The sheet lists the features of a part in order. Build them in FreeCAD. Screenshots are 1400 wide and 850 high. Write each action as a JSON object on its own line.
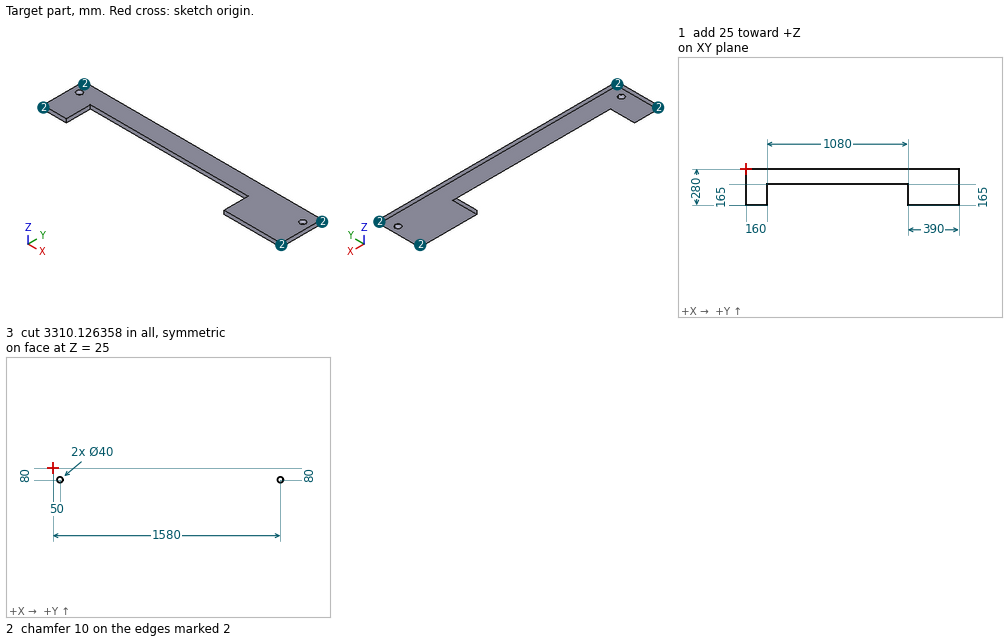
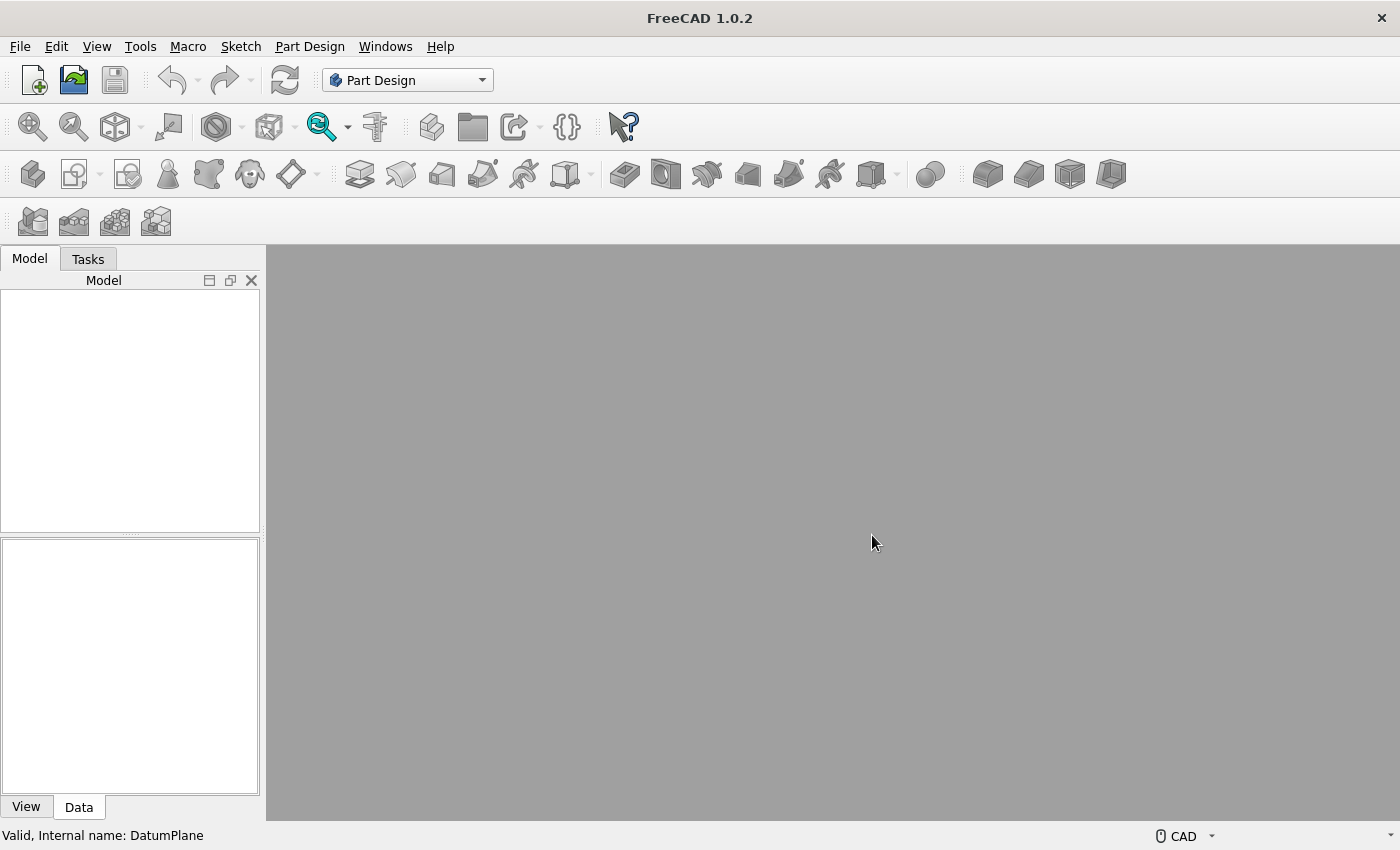
{"action": "key", "text": "ctrl+n"}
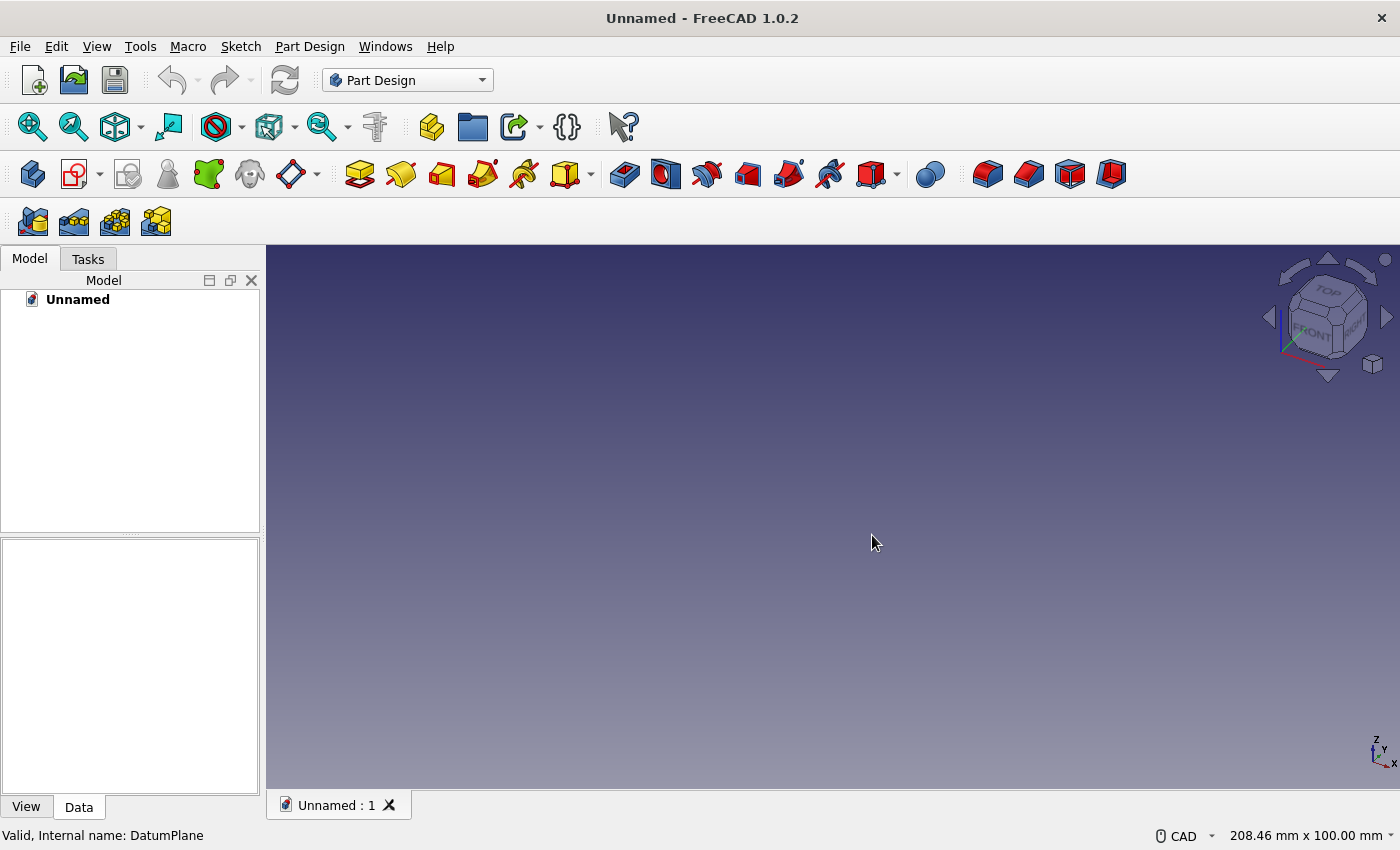
{"action": "left_click", "coordinate": [74, 174]}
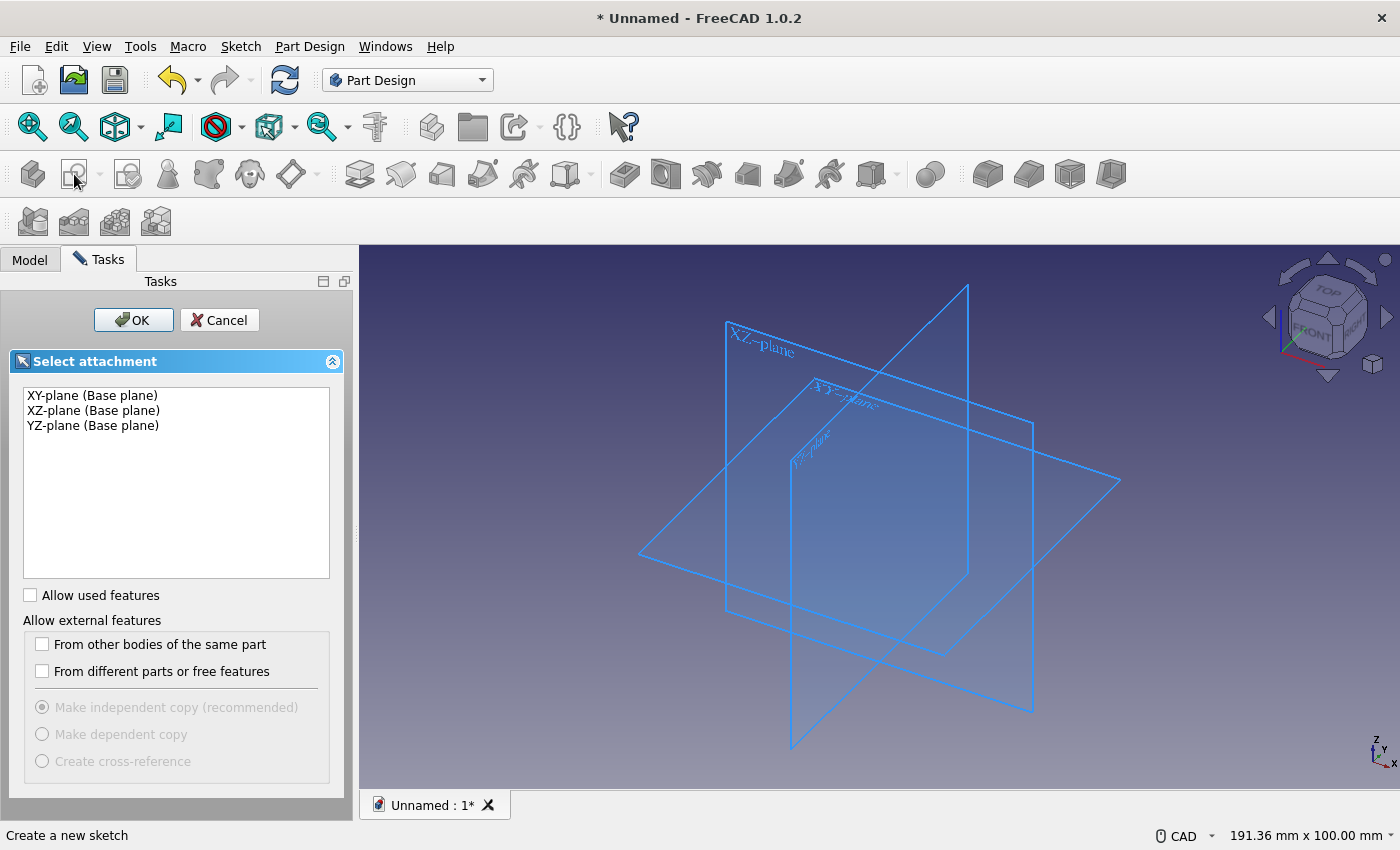
{"action": "left_click", "coordinate": [84, 396]}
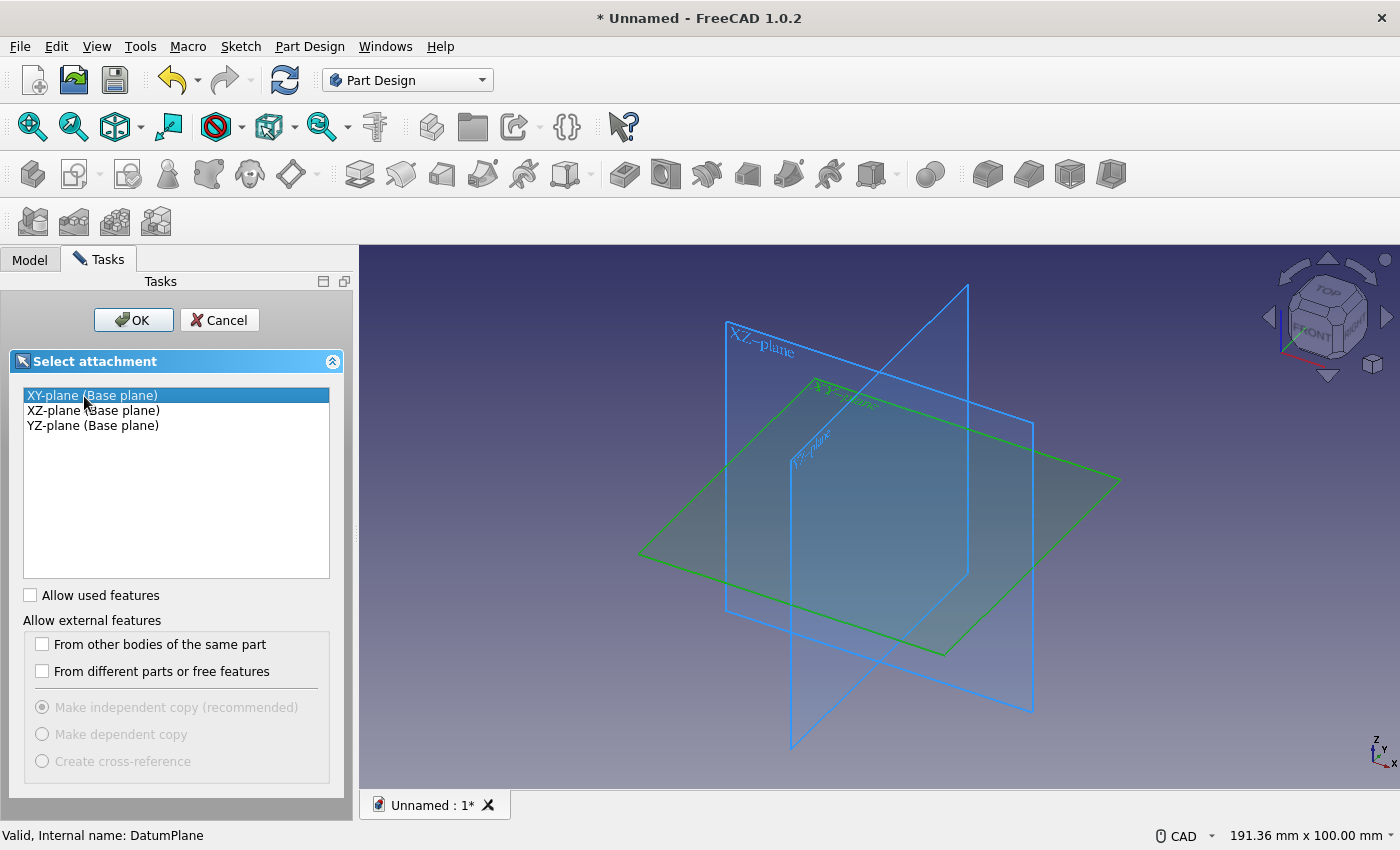
{"action": "left_click", "coordinate": [134, 320]}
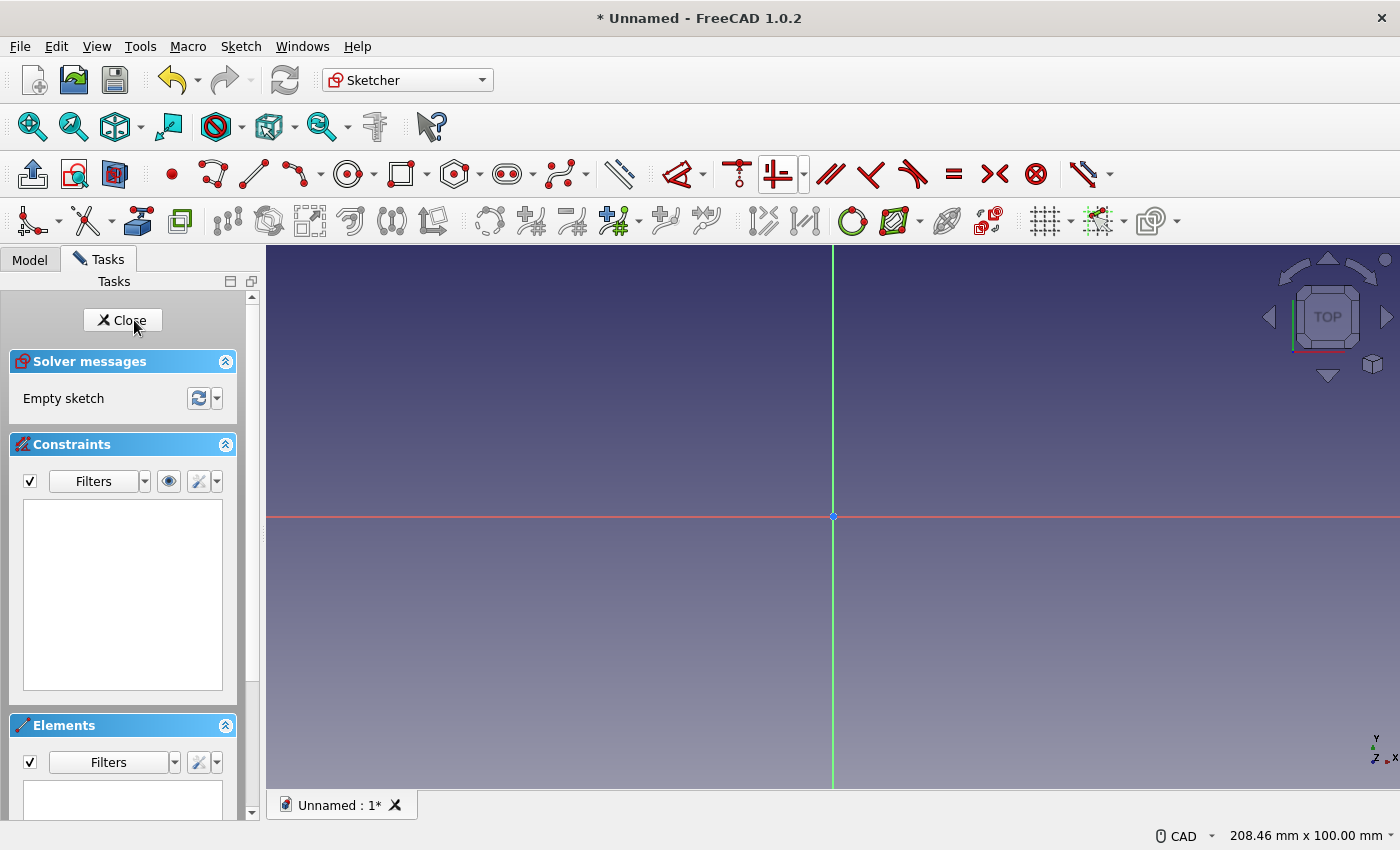
{"action": "scroll", "coordinate": [403, 456], "scroll_direction": "down", "scroll_amount": 13}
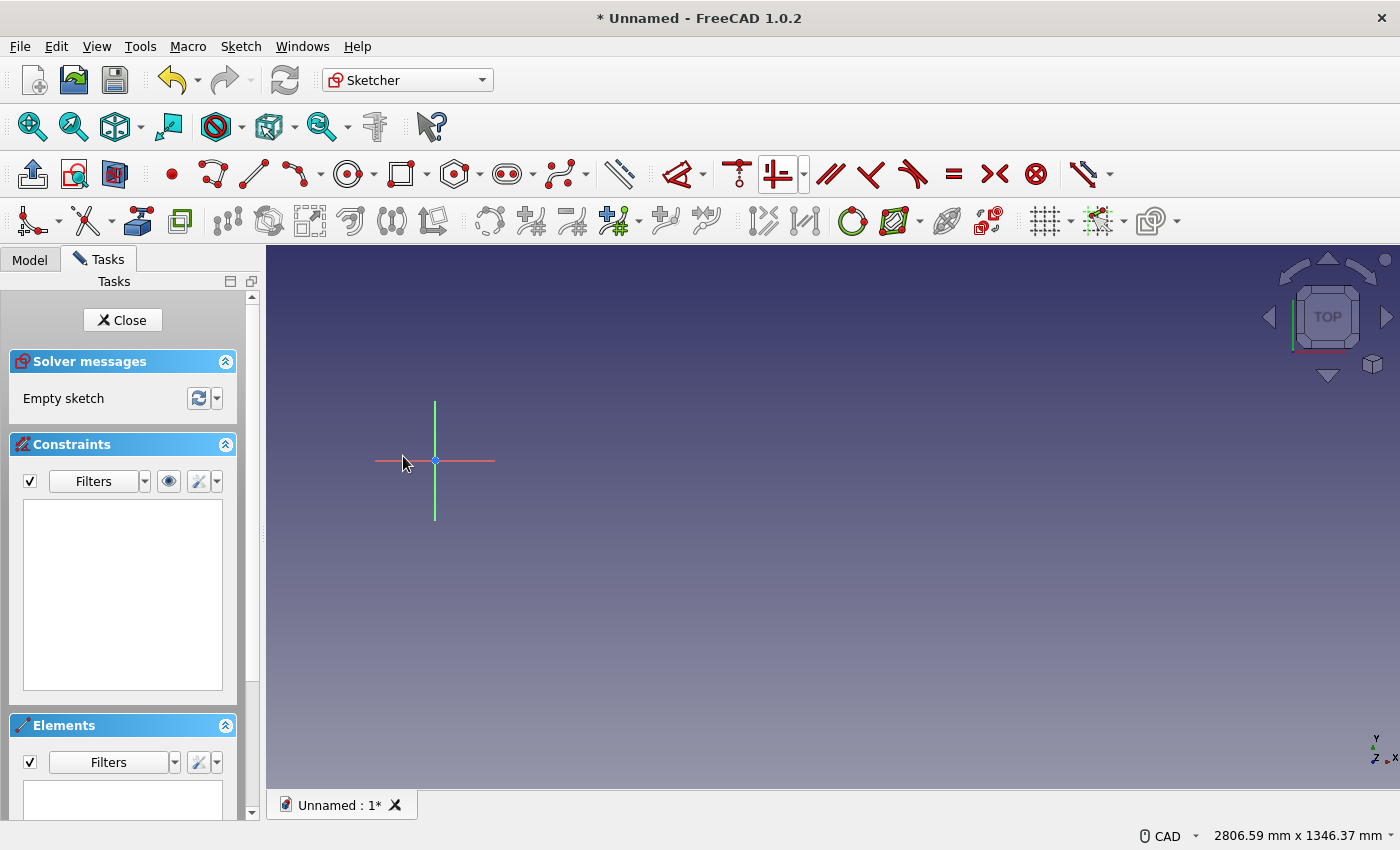
{"action": "key", "text": "g m"}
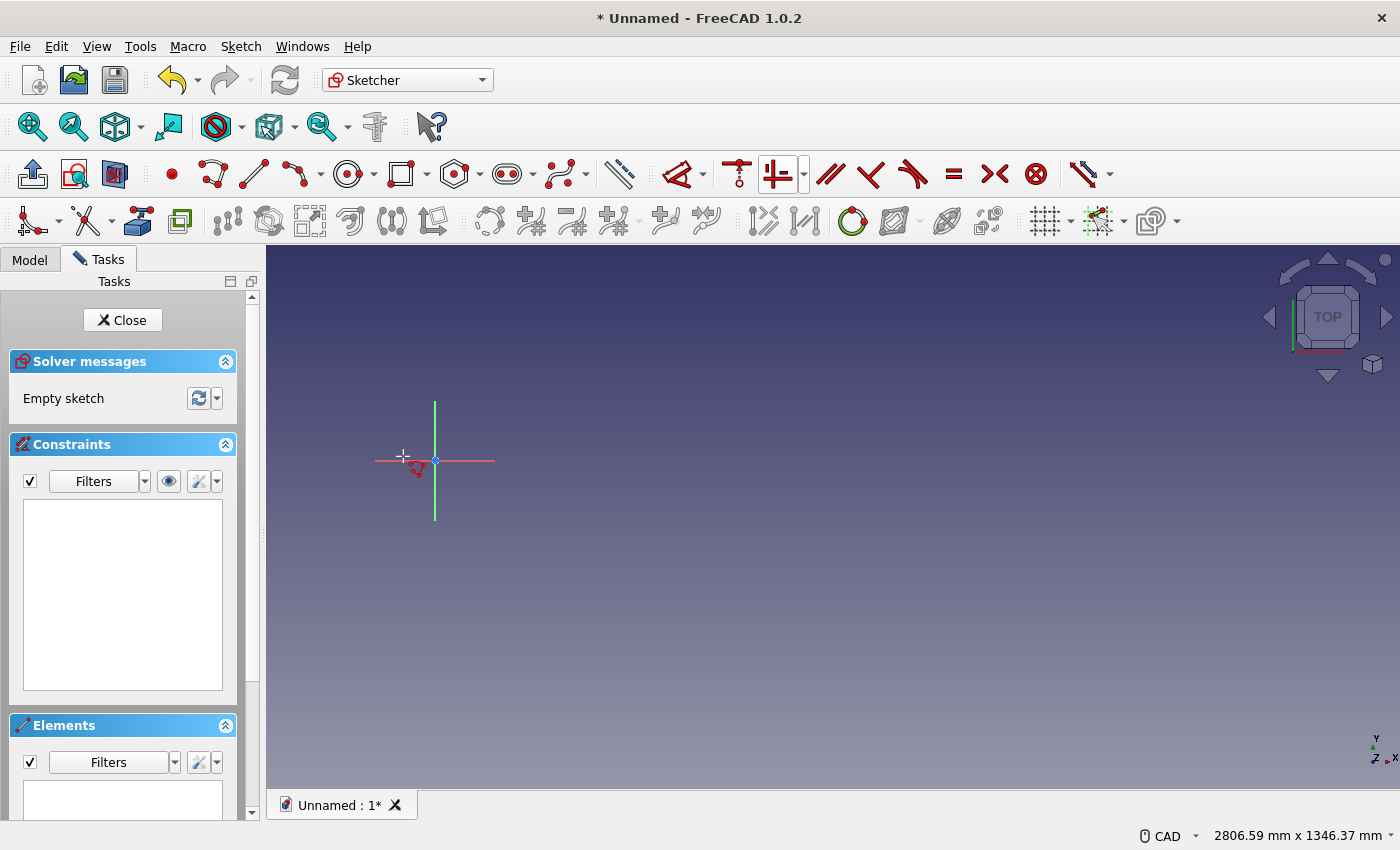
{"action": "left_click", "coordinate": [435, 461]}
{"action": "left_click", "coordinate": [444, 574]}
{"action": "left_click", "coordinate": [500, 574]}
{"action": "left_click", "coordinate": [500, 507]}
{"action": "left_click", "coordinate": [936, 507]}
{"action": "left_click", "coordinate": [936, 574]}
{"action": "left_click", "coordinate": [1094, 574]}
{"action": "left_click", "coordinate": [1094, 470]}
{"action": "left_click", "coordinate": [435, 461]}
{"action": "key", "text": "Escape"}
{"action": "key", "text": "Escape"}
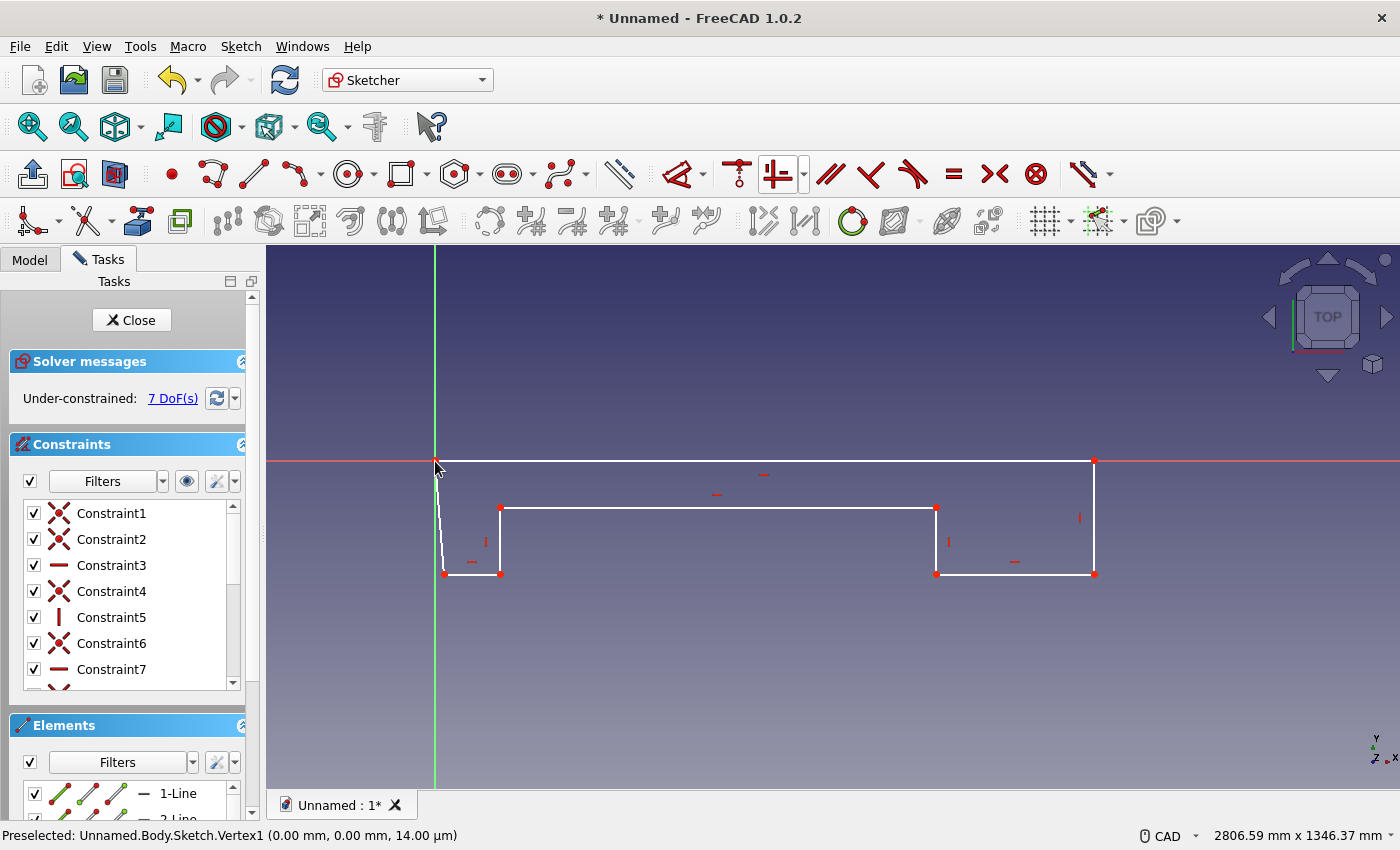
{"action": "left_click", "coordinate": [438, 495]}